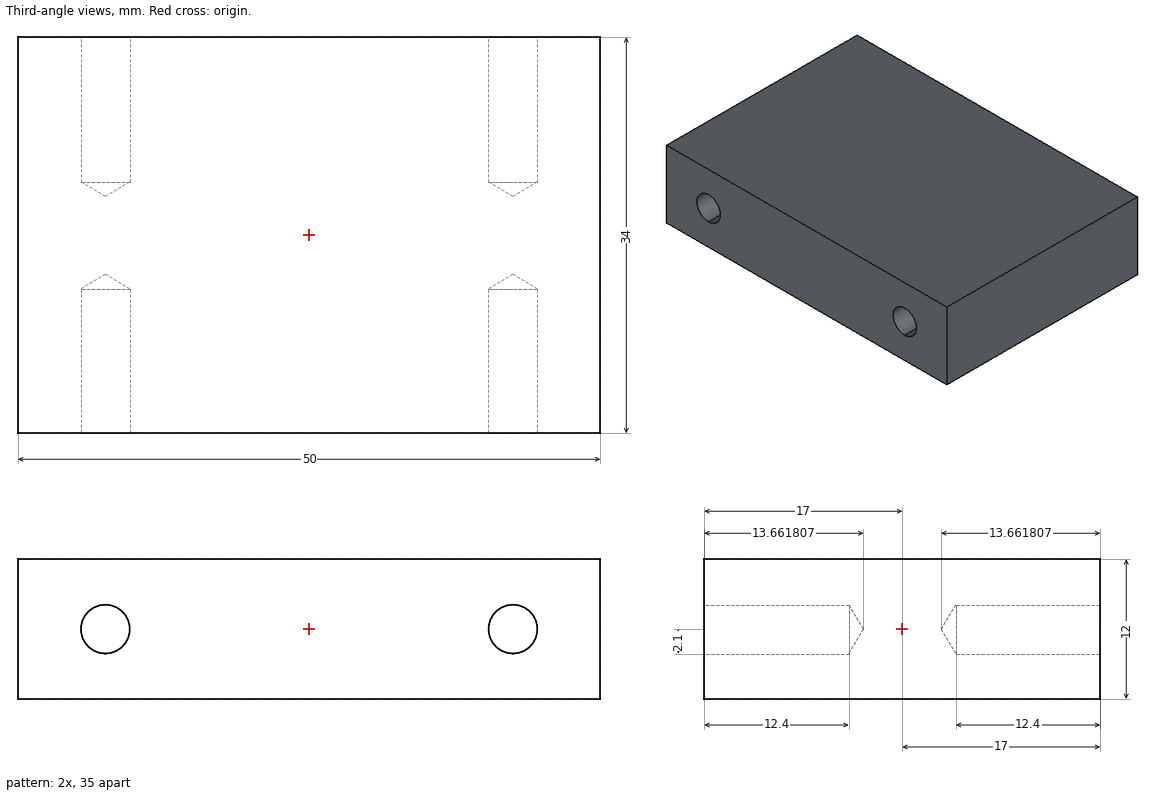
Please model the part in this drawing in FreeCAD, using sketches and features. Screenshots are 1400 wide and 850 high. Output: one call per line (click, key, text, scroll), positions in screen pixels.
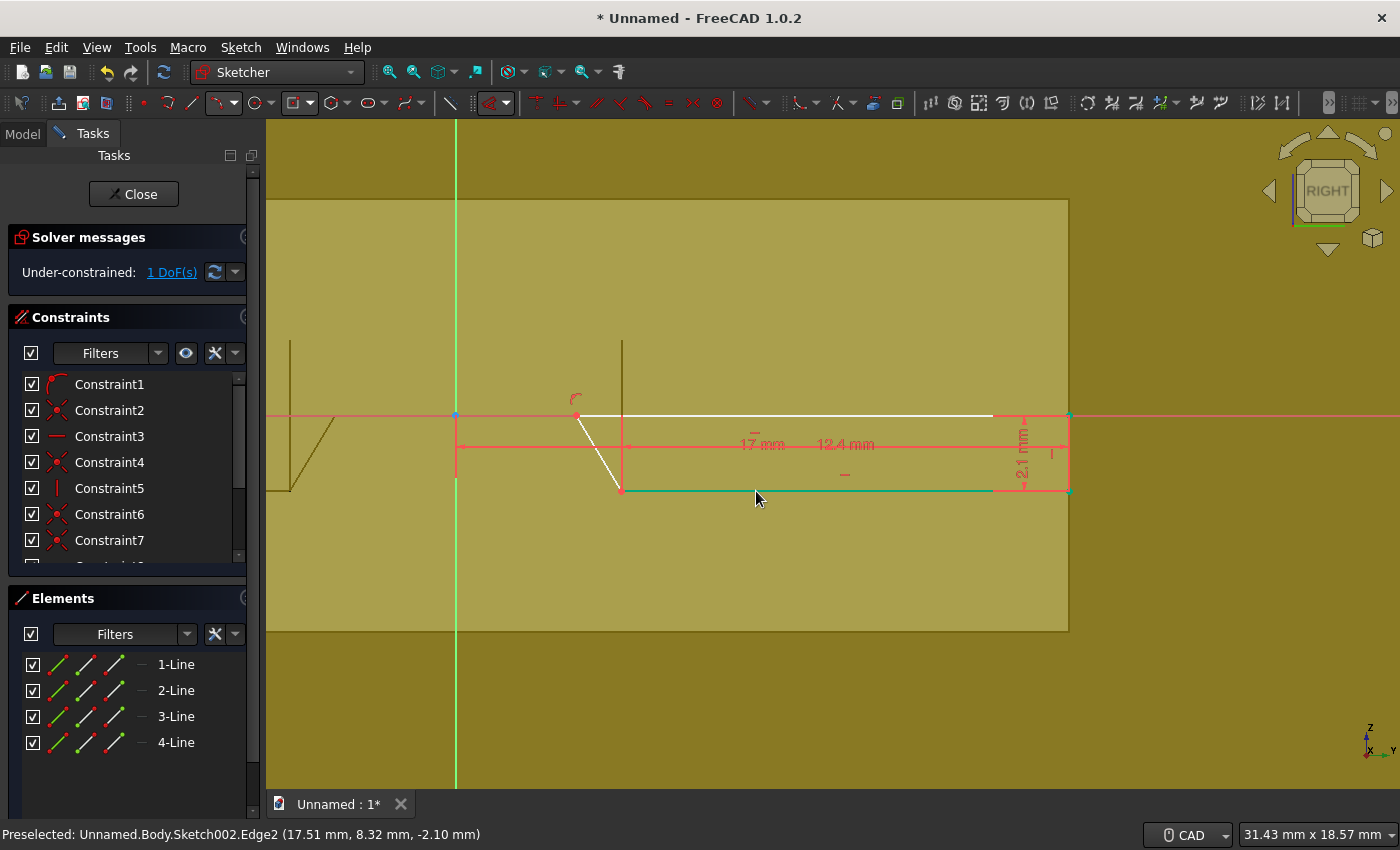
click(921, 416)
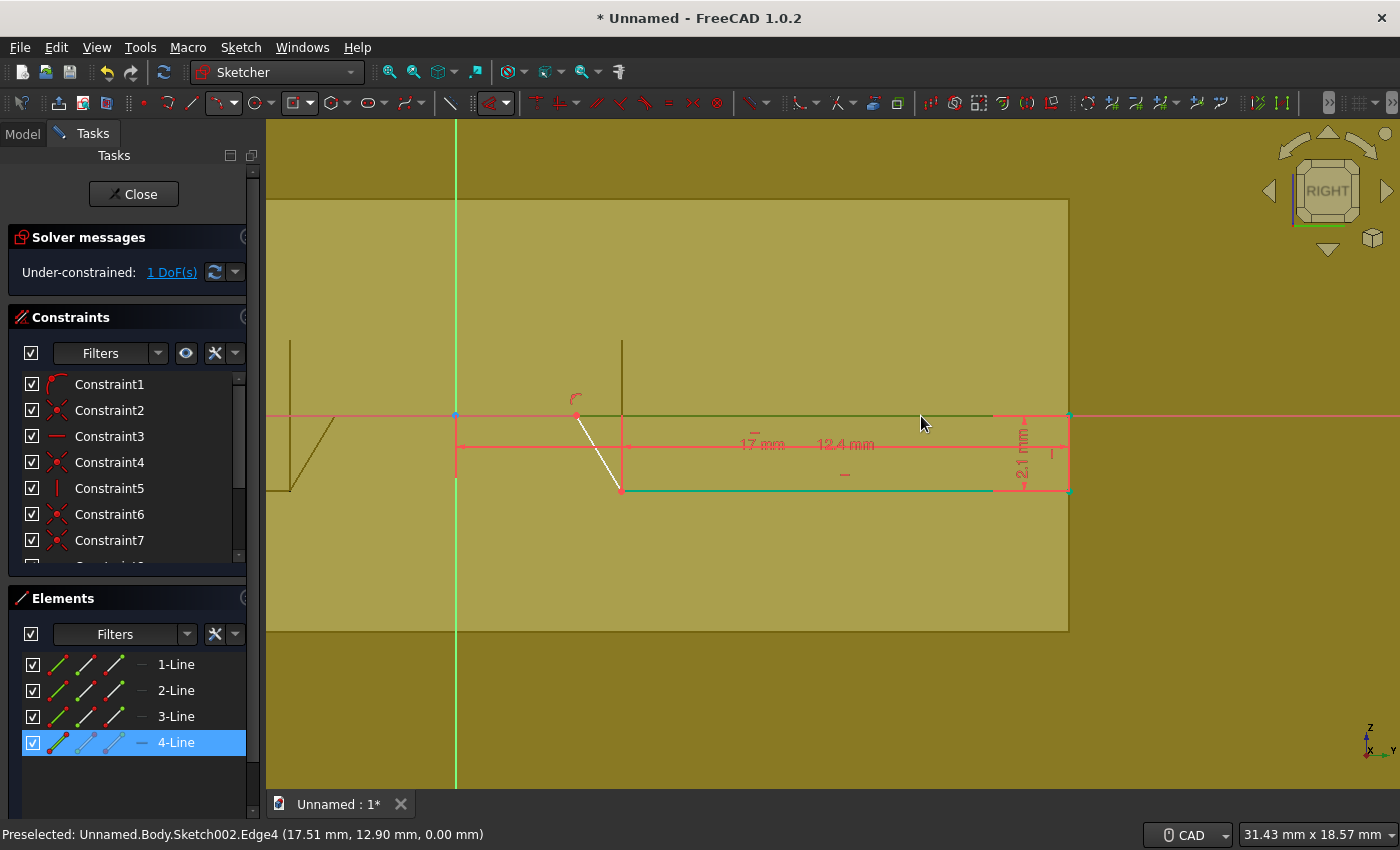
key(l)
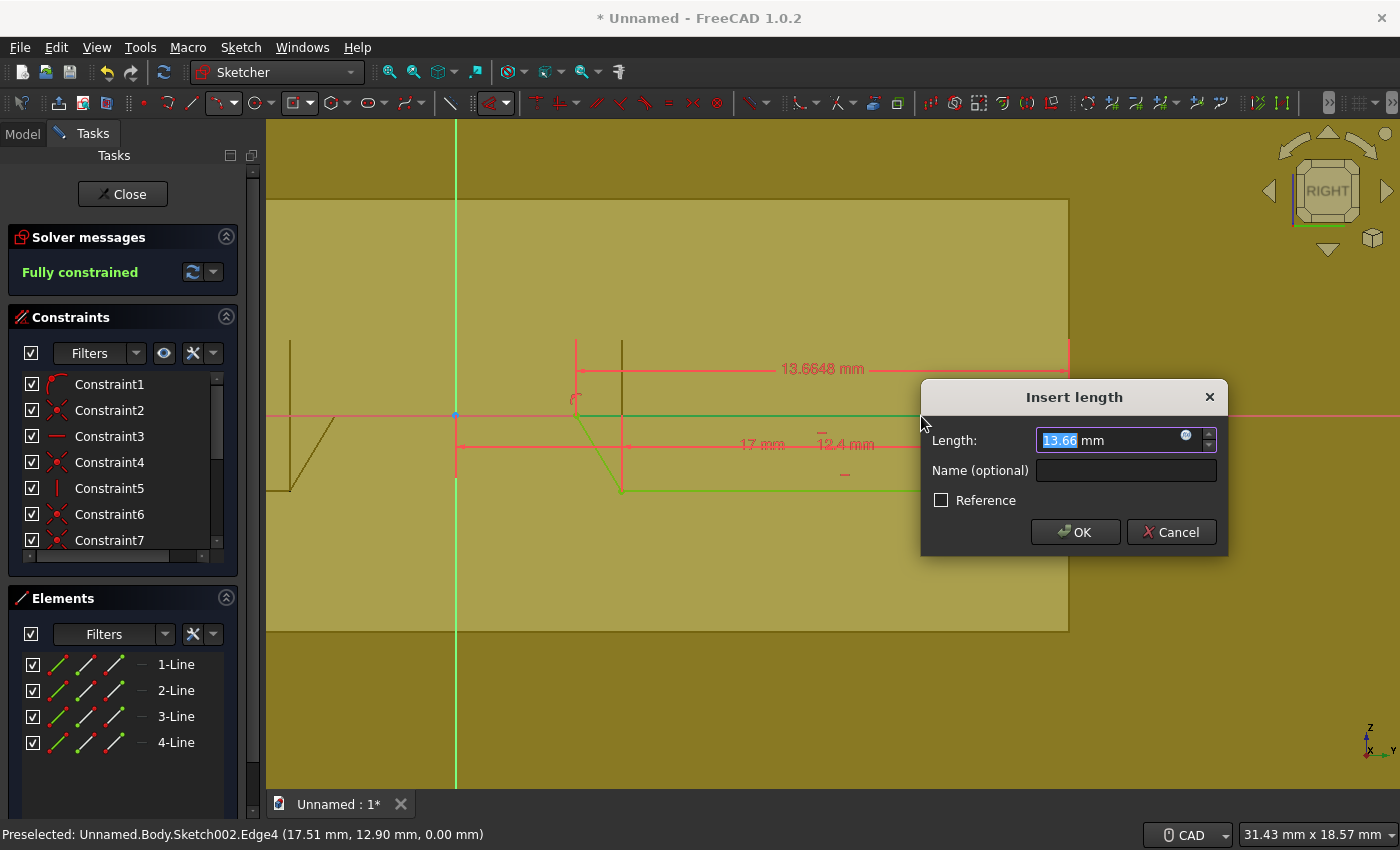
text(13.661807)
key(Return)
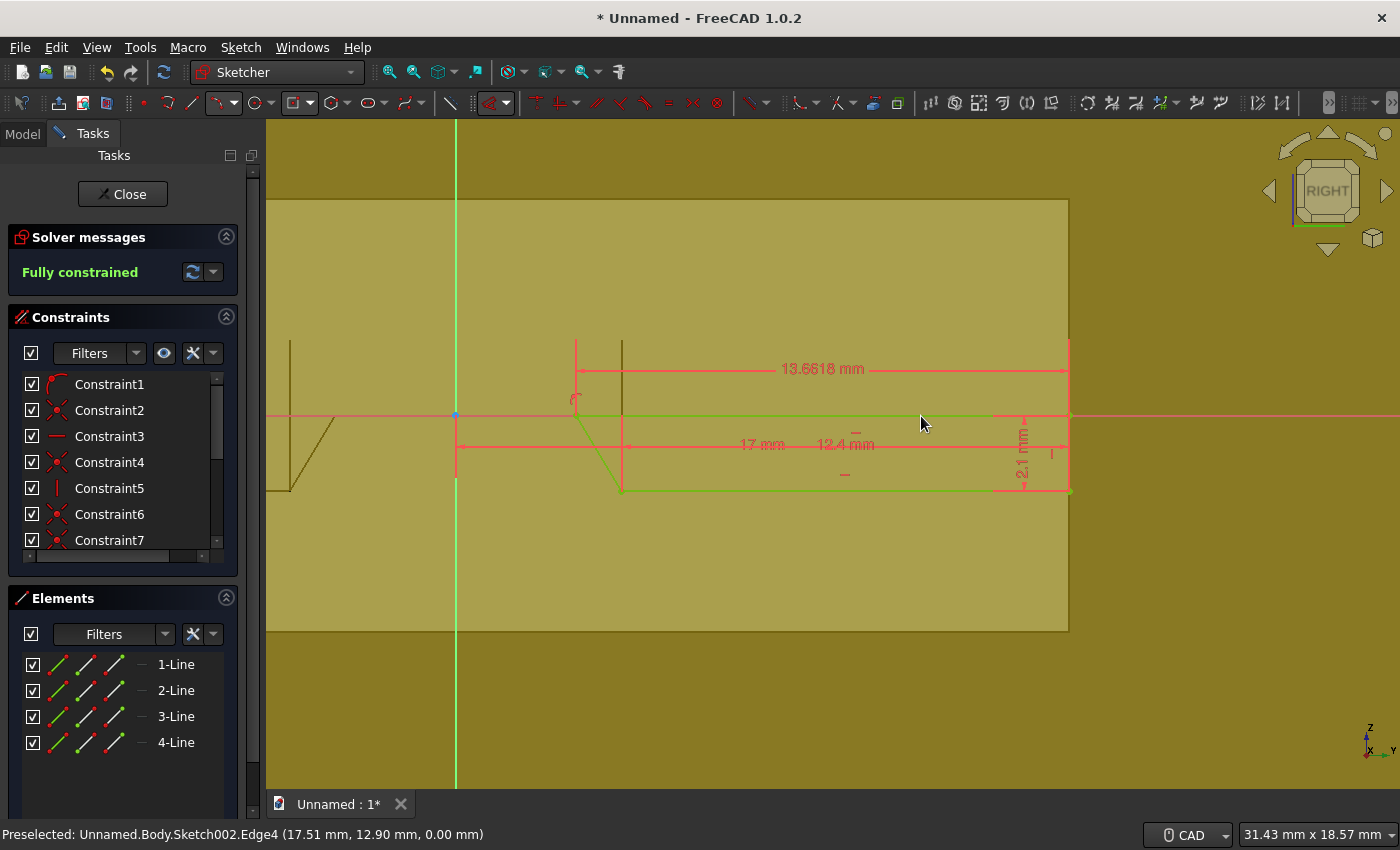
click(123, 194)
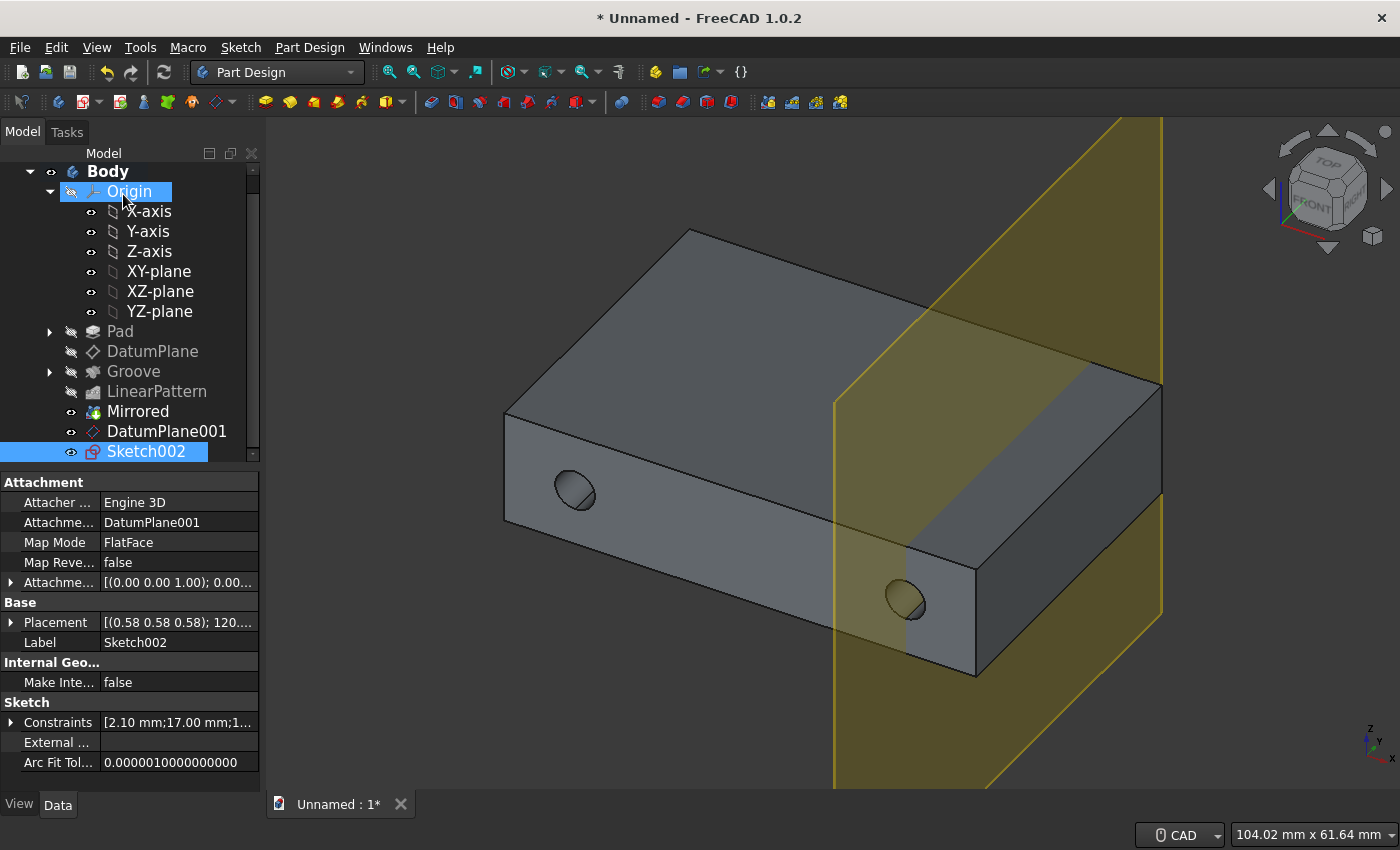
click(480, 102)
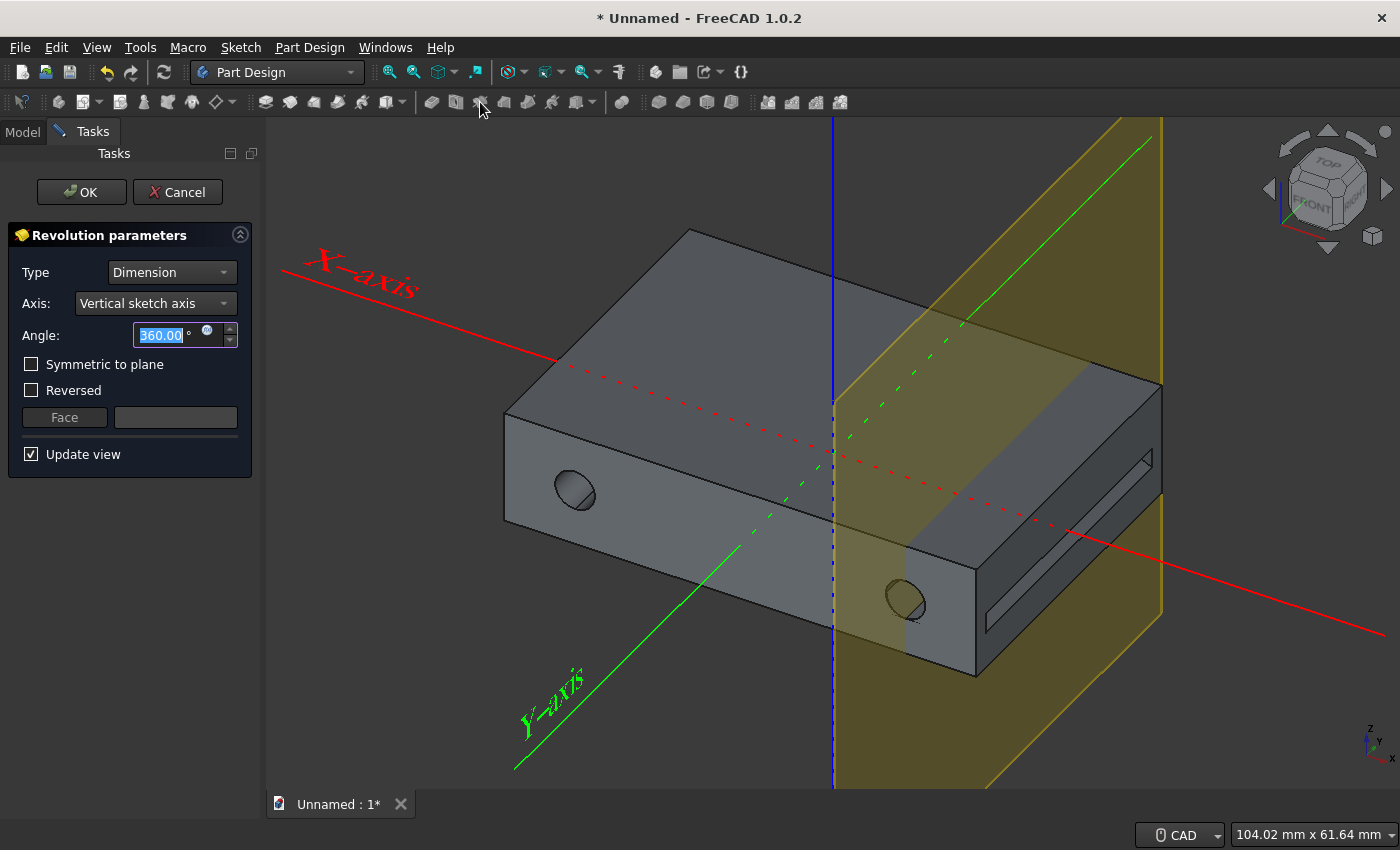
click(156, 304)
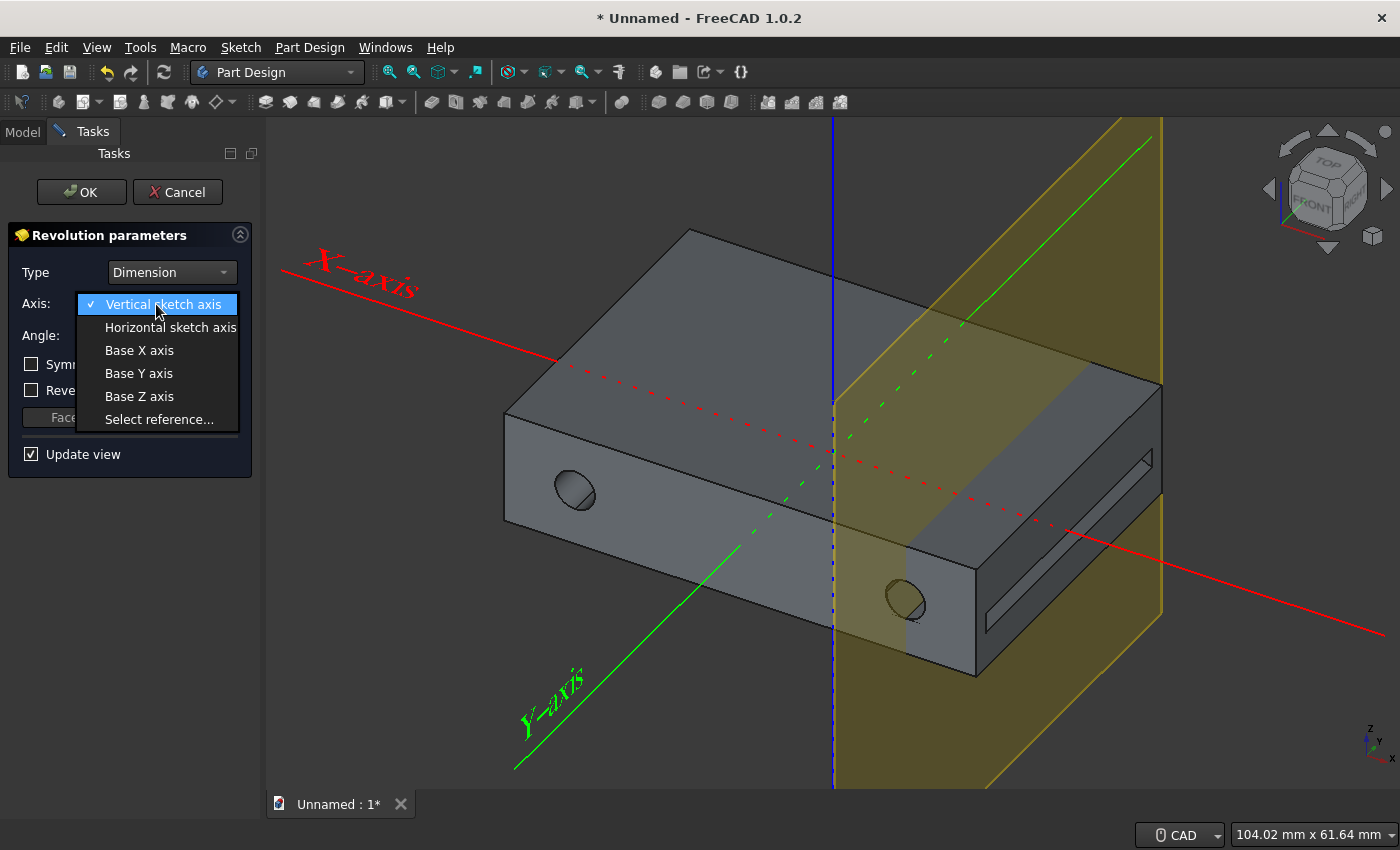
click(156, 328)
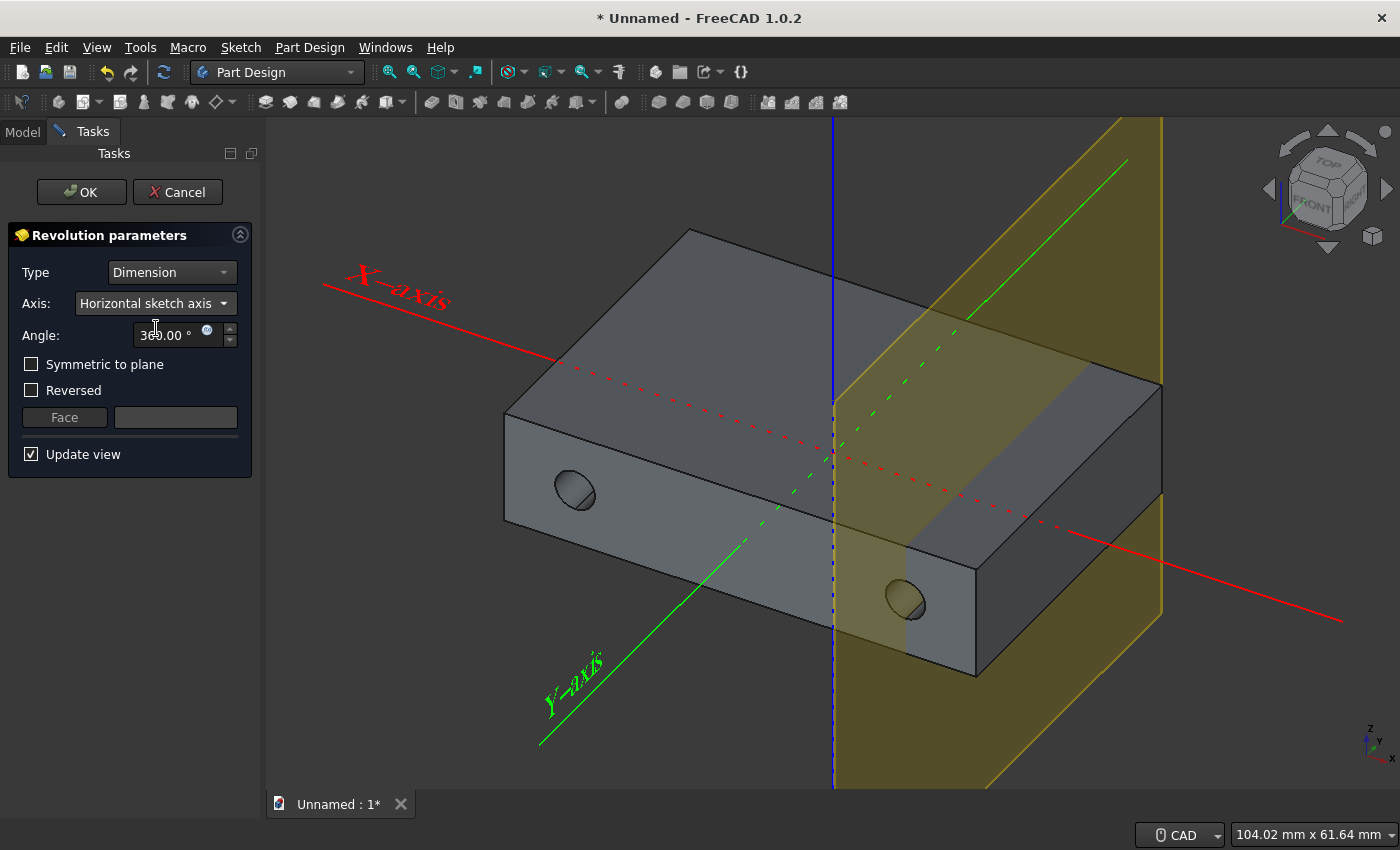
click(82, 192)